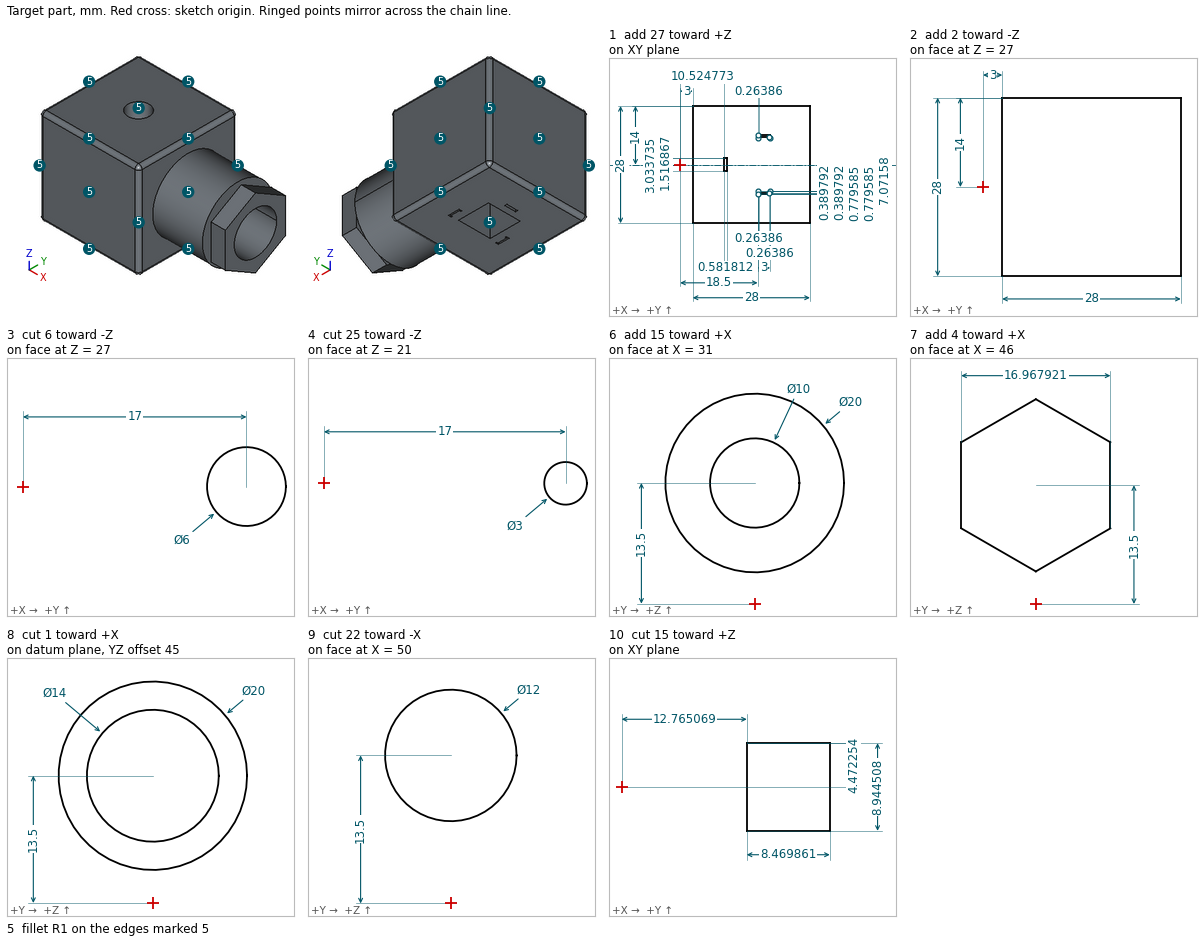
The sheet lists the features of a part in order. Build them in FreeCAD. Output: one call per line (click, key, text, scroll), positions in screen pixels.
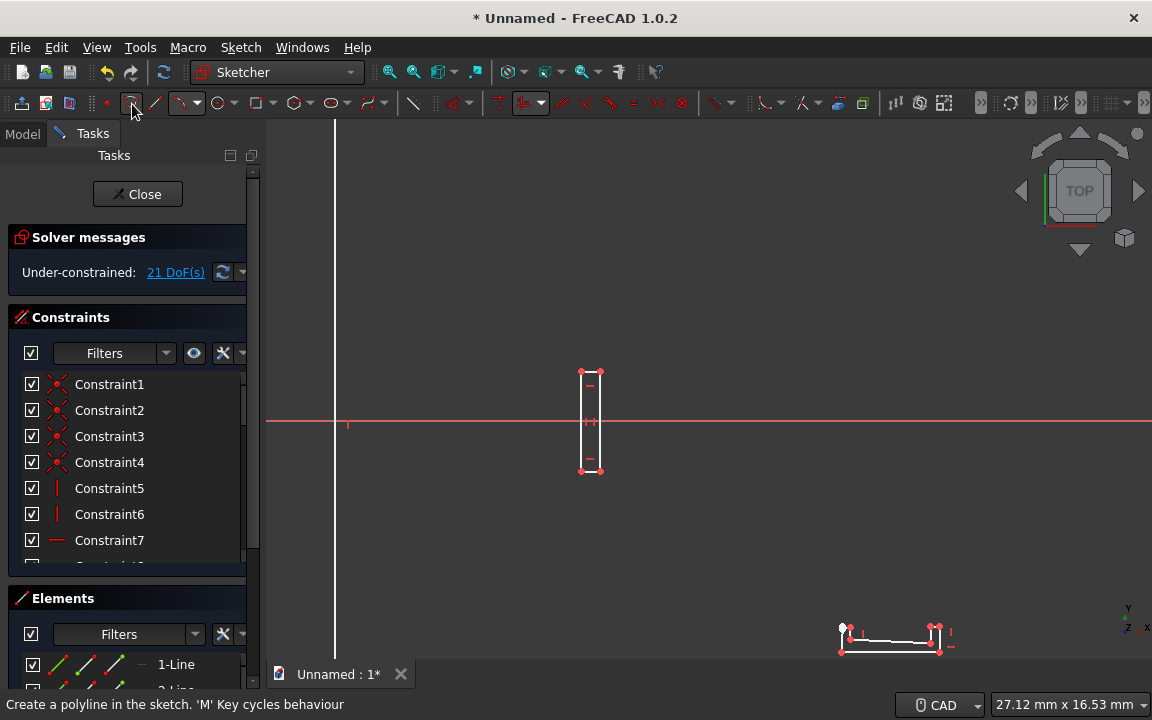
click(842, 215)
click(842, 190)
click(940, 190)
click(940, 215)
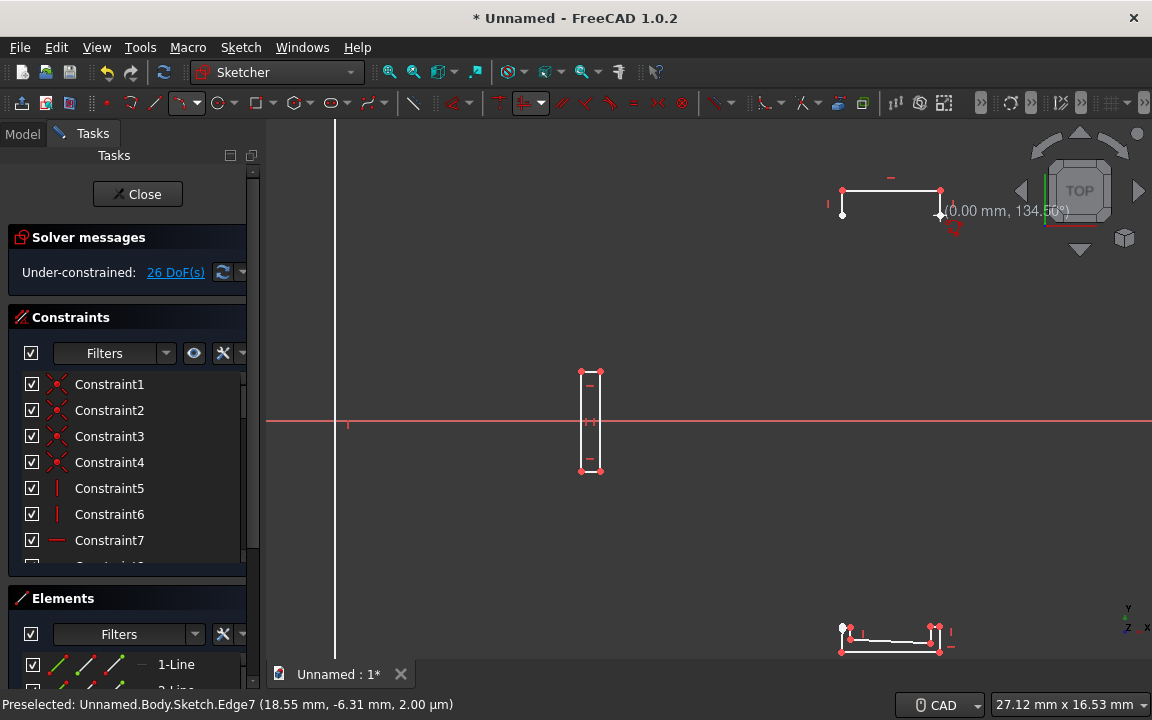
scroll(931, 215, up, 4)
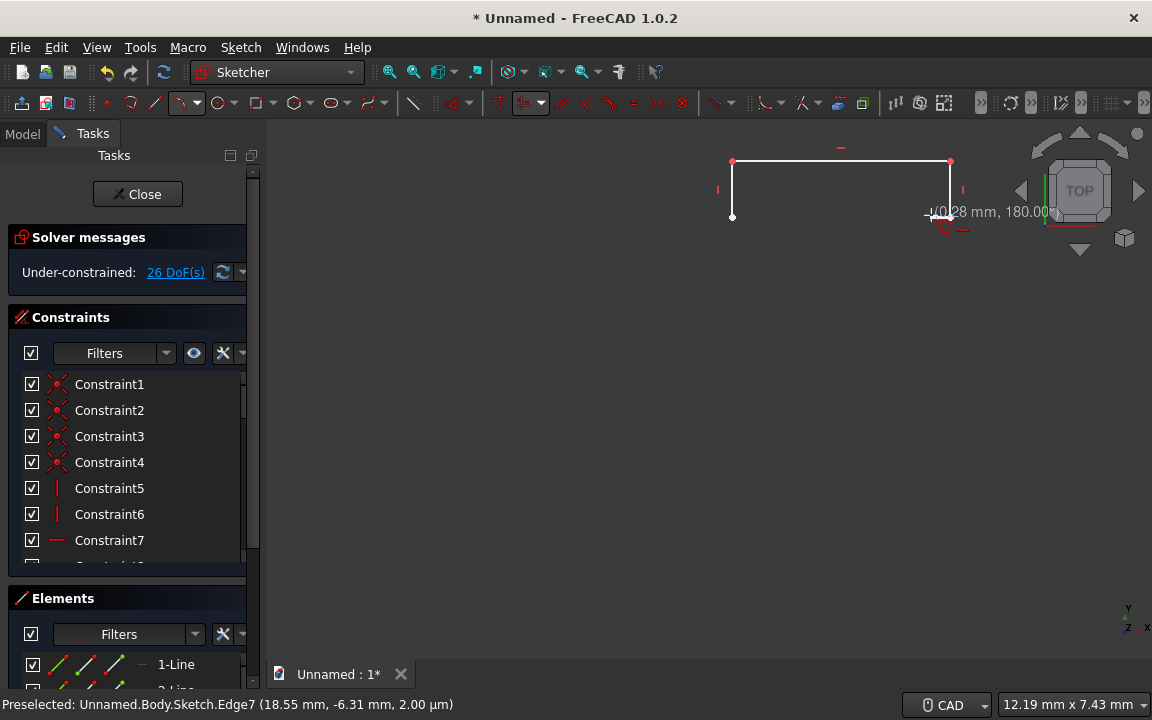
click(930, 215)
click(930, 187)
click(750, 187)
click(750, 216)
click(732, 217)
key(Escape)
key(Escape)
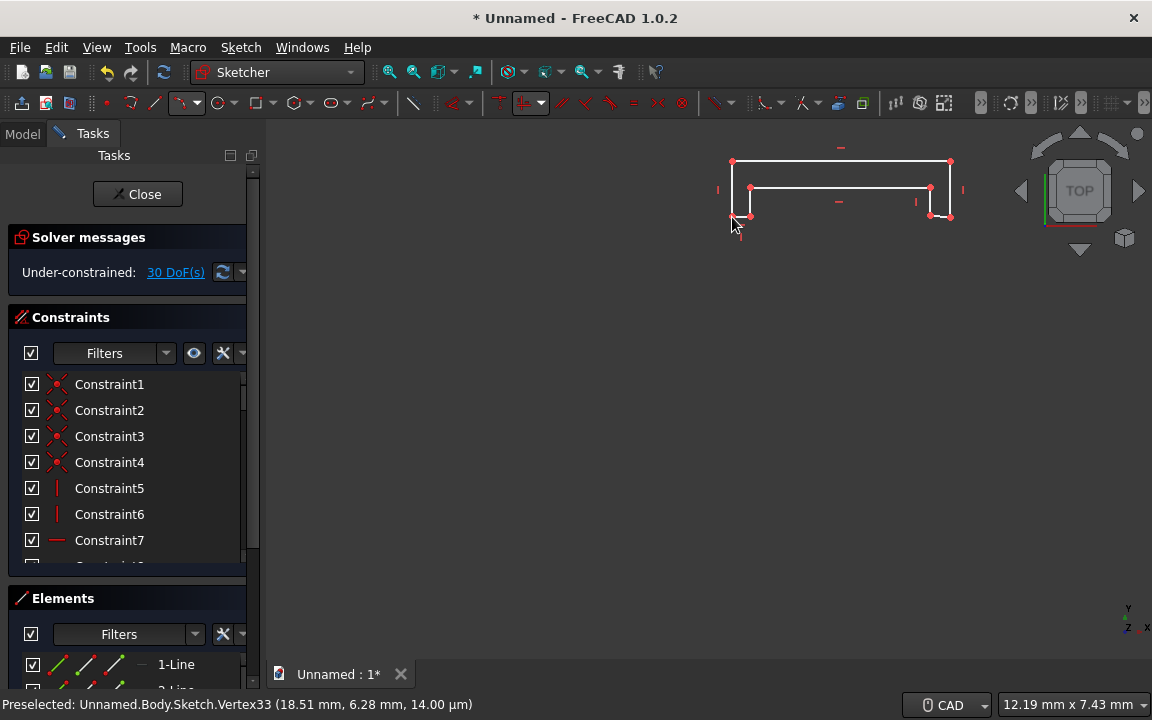
scroll(666, 333, down, 9)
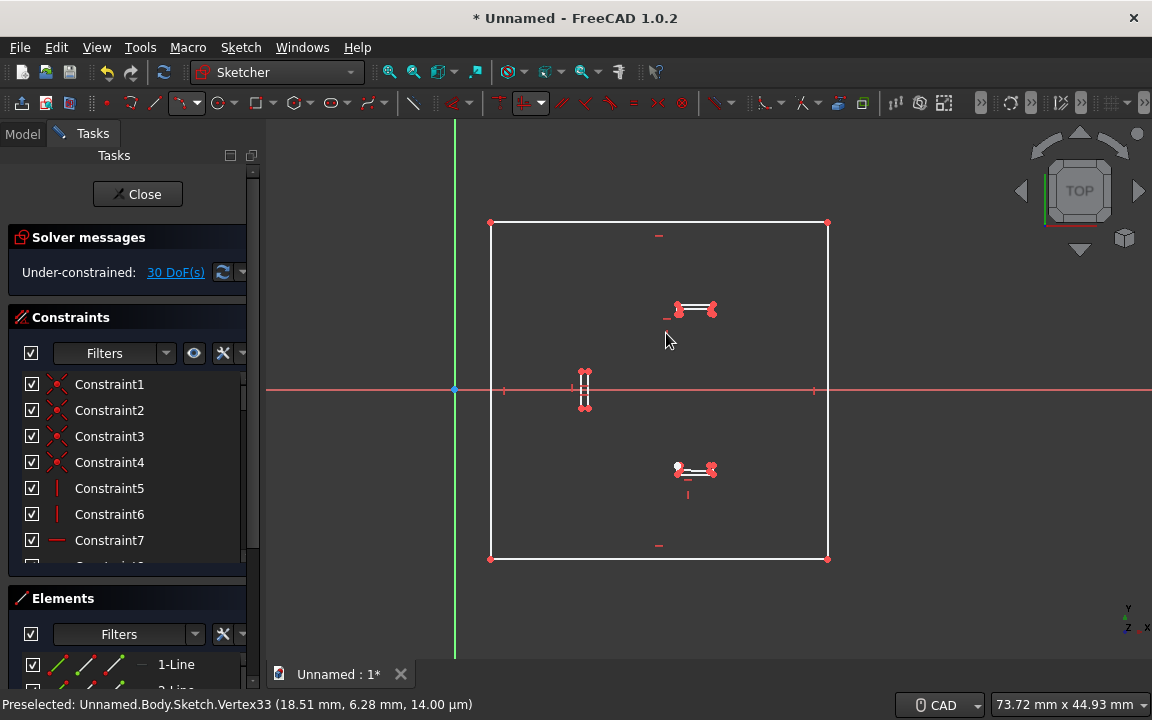
scroll(679, 466, up, 12)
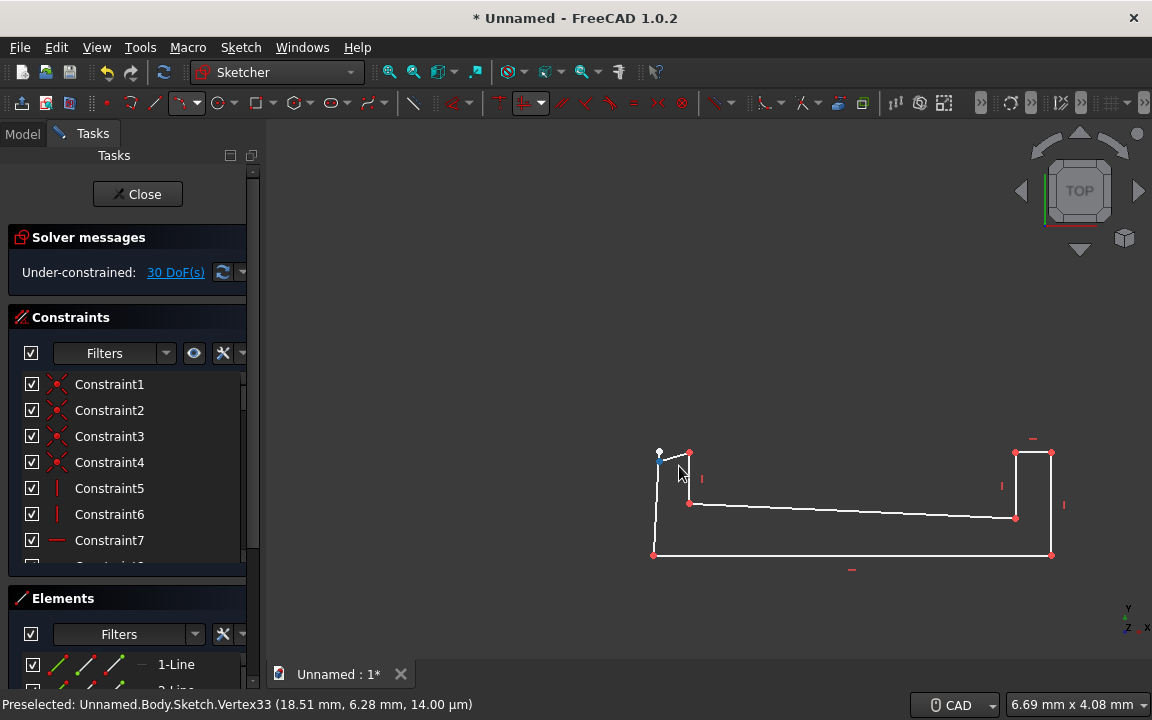
click(674, 457)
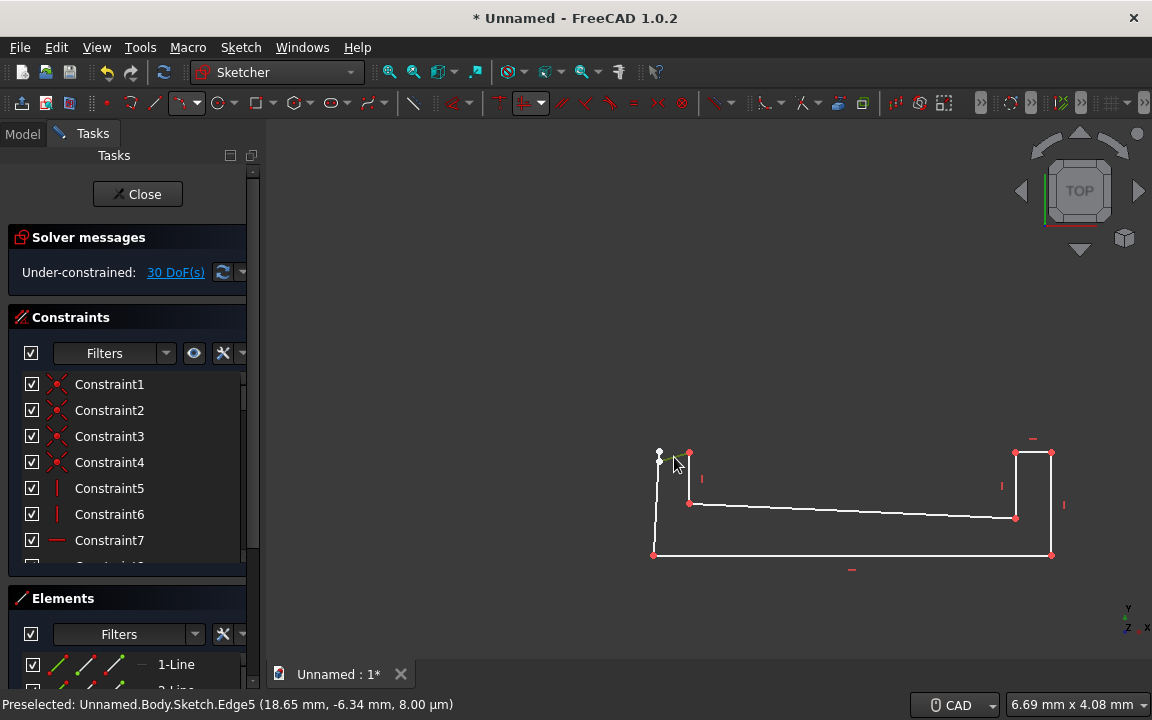
click(544, 104)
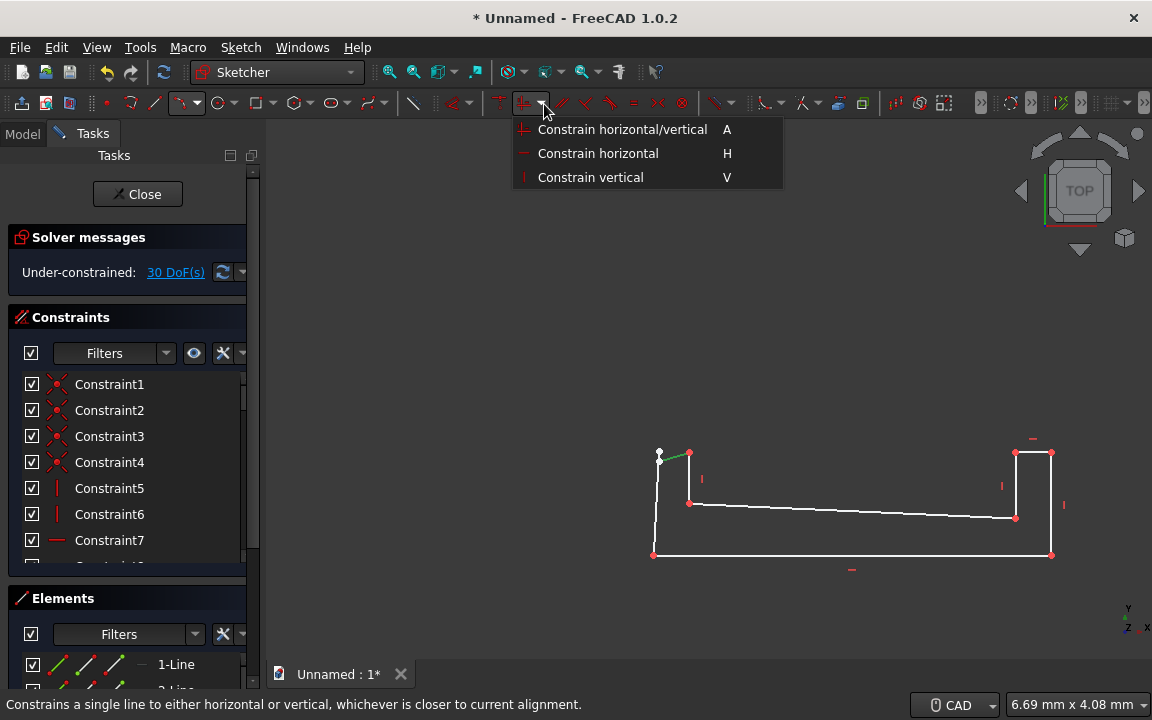
click(648, 153)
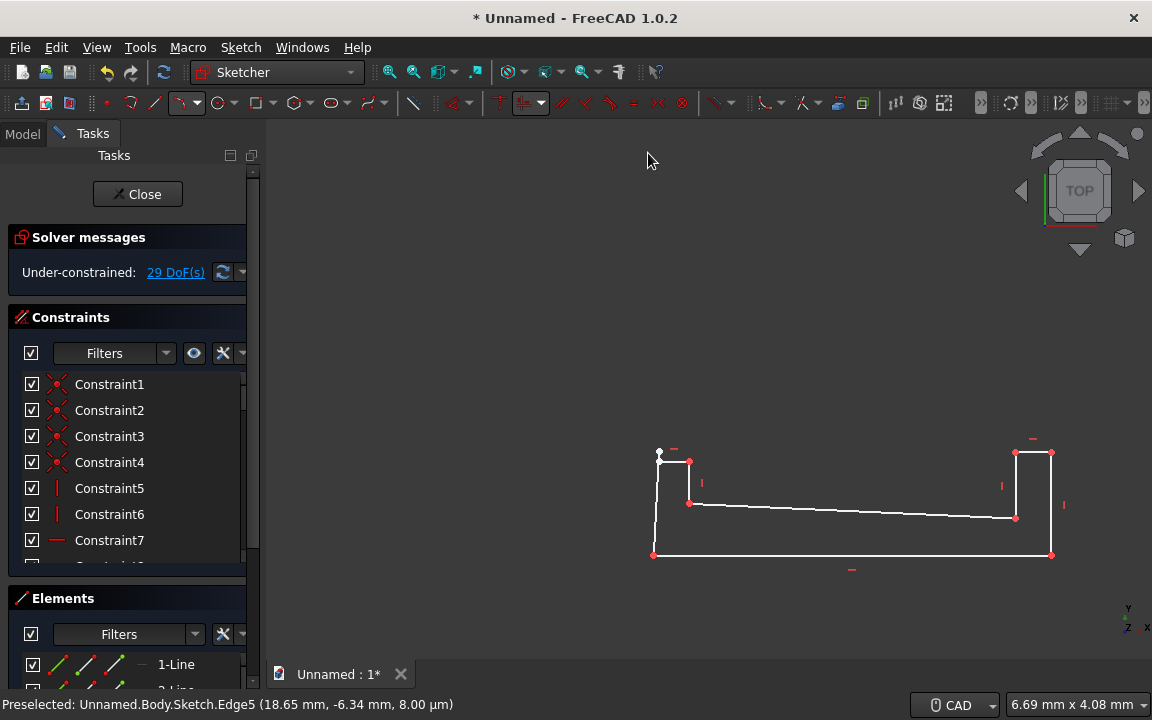
scroll(679, 466, down, 12)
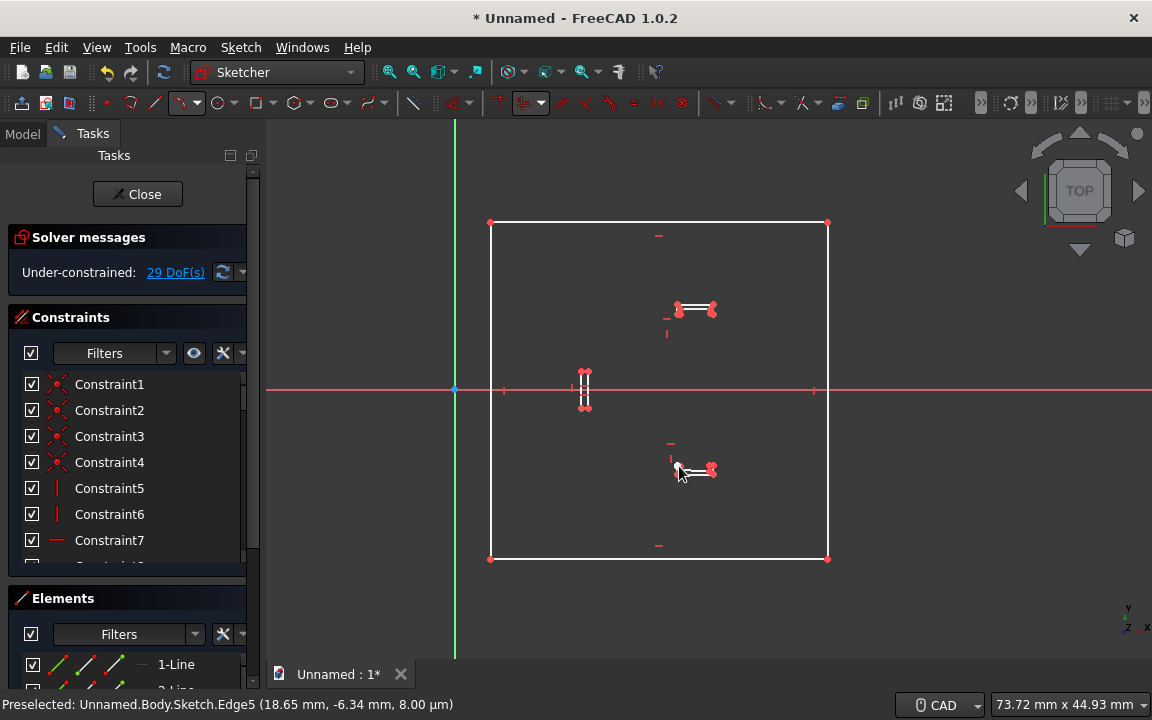
scroll(689, 470, up, 6)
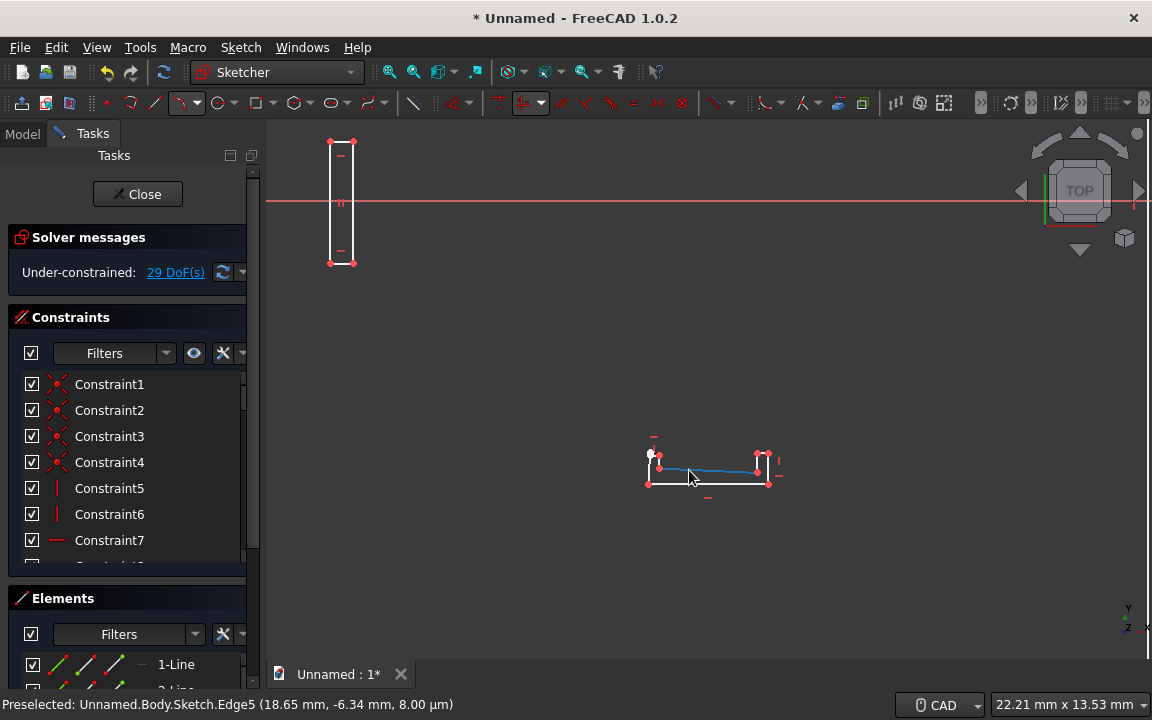
click(689, 470)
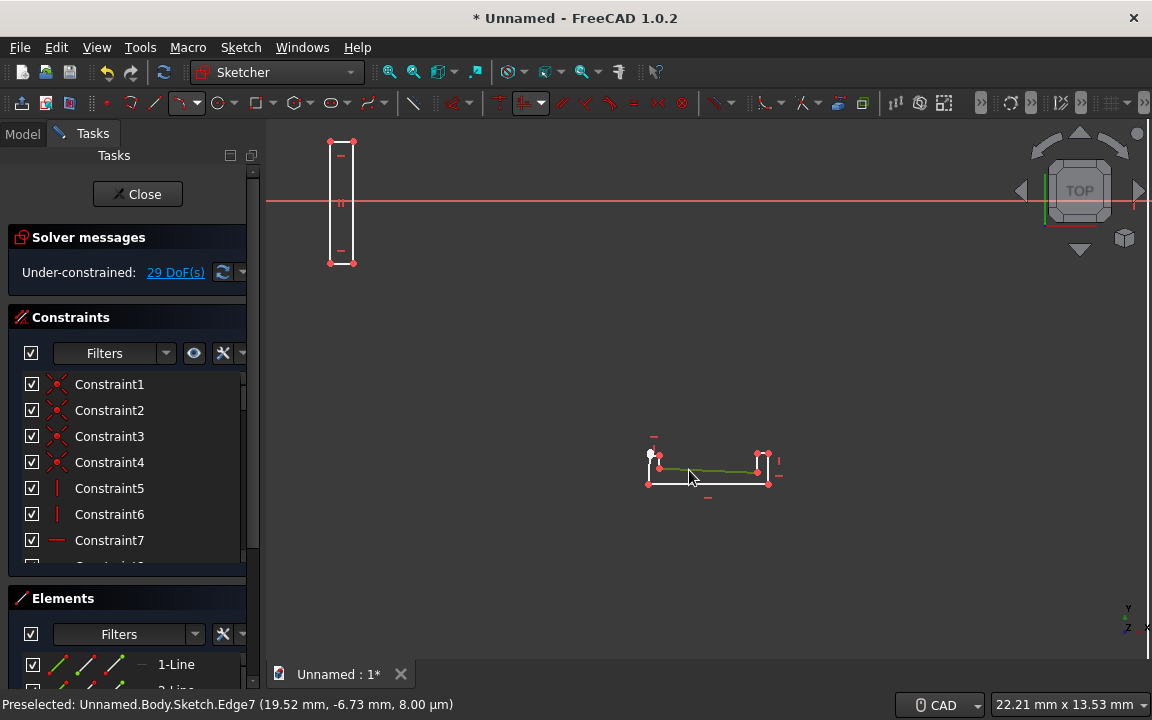
key(h)